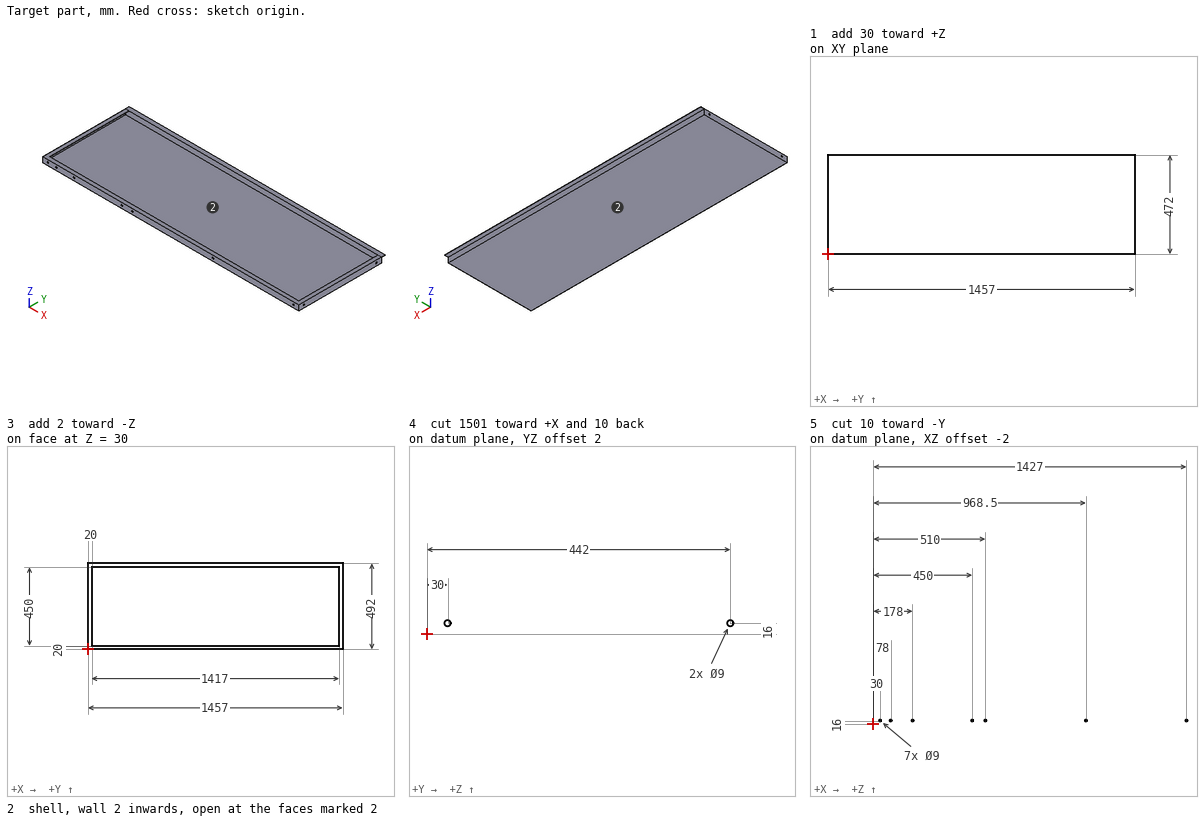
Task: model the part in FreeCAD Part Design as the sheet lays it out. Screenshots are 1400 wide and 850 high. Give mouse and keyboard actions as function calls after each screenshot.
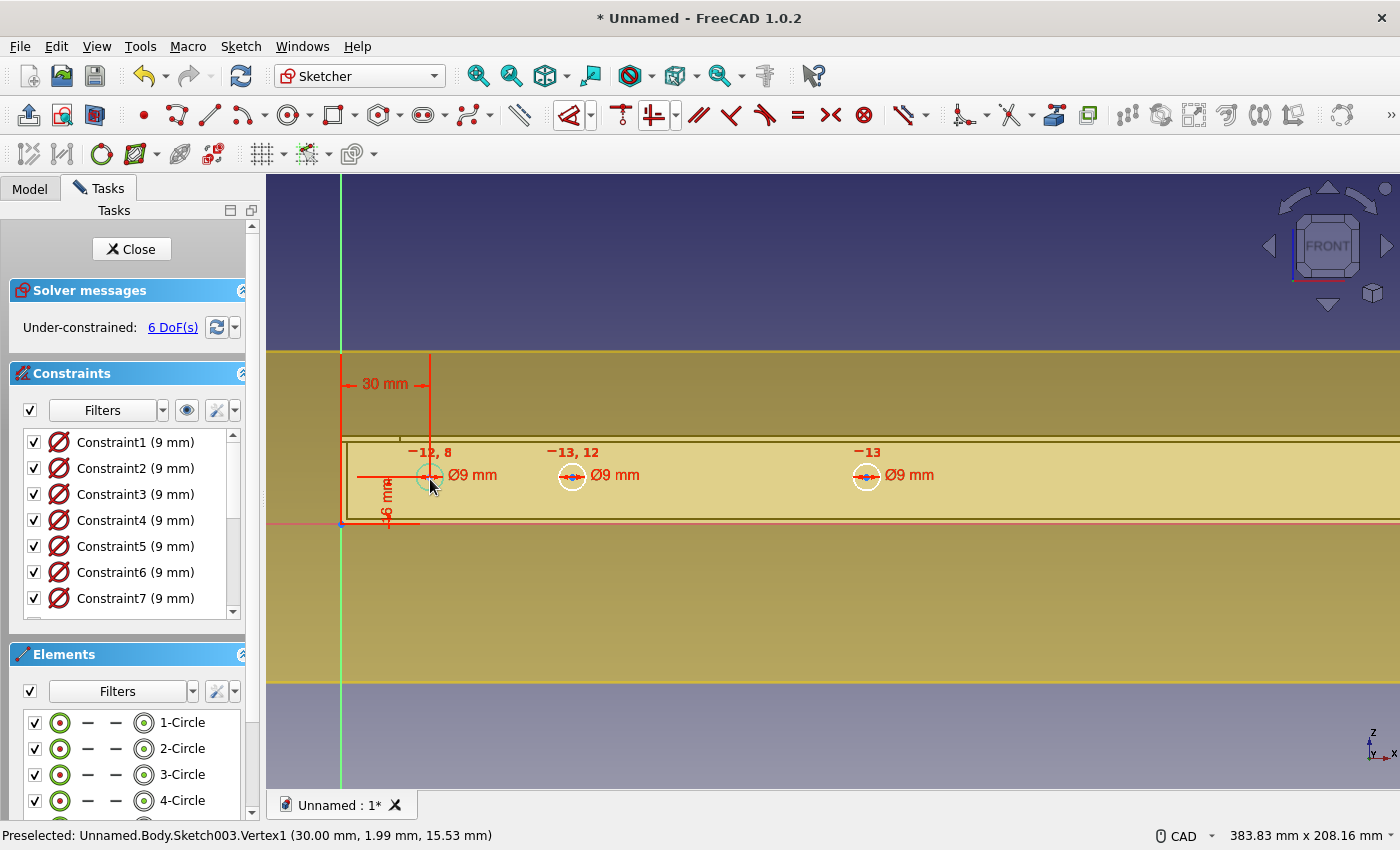
scroll(430, 479, down, 9)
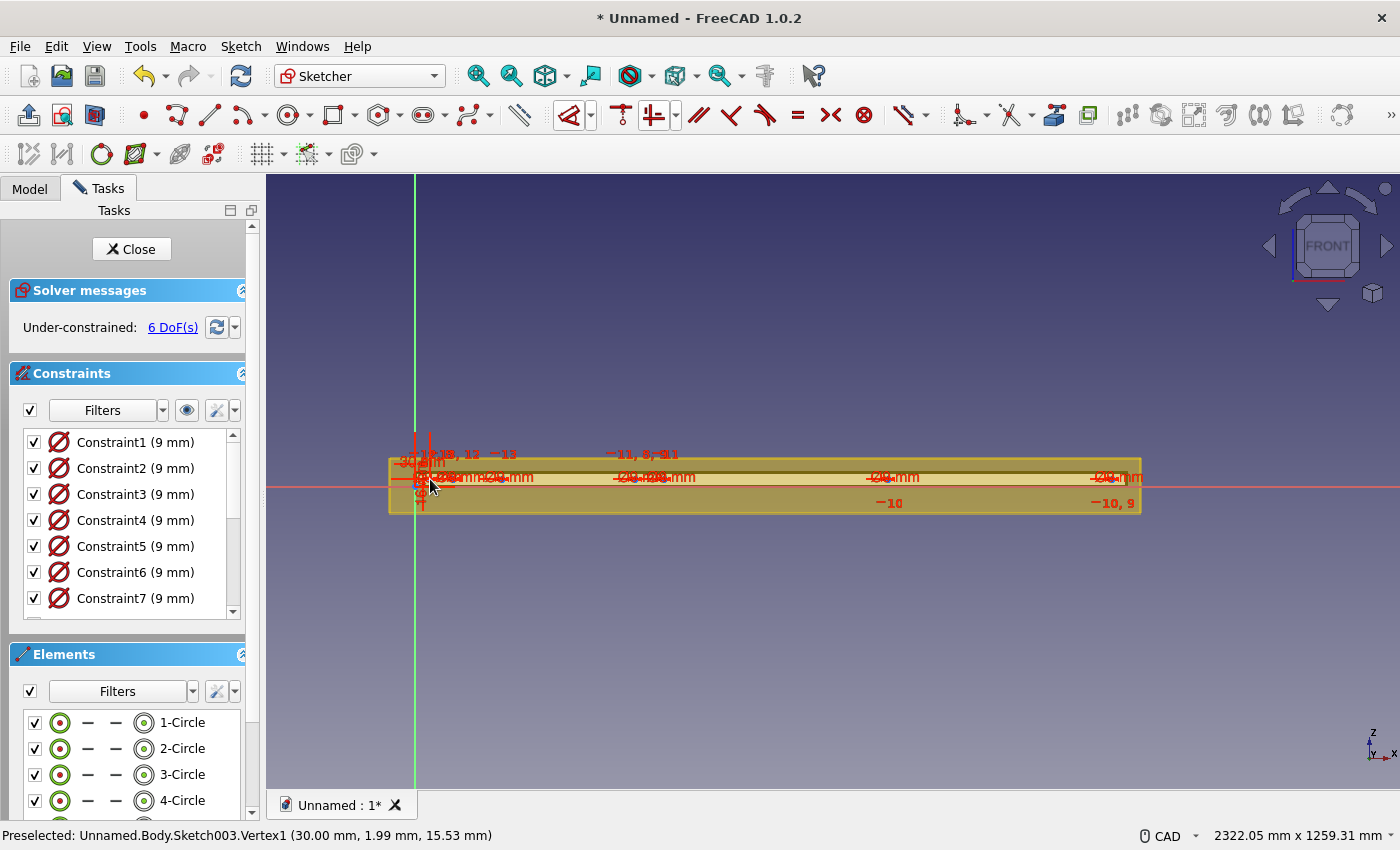
click(454, 479)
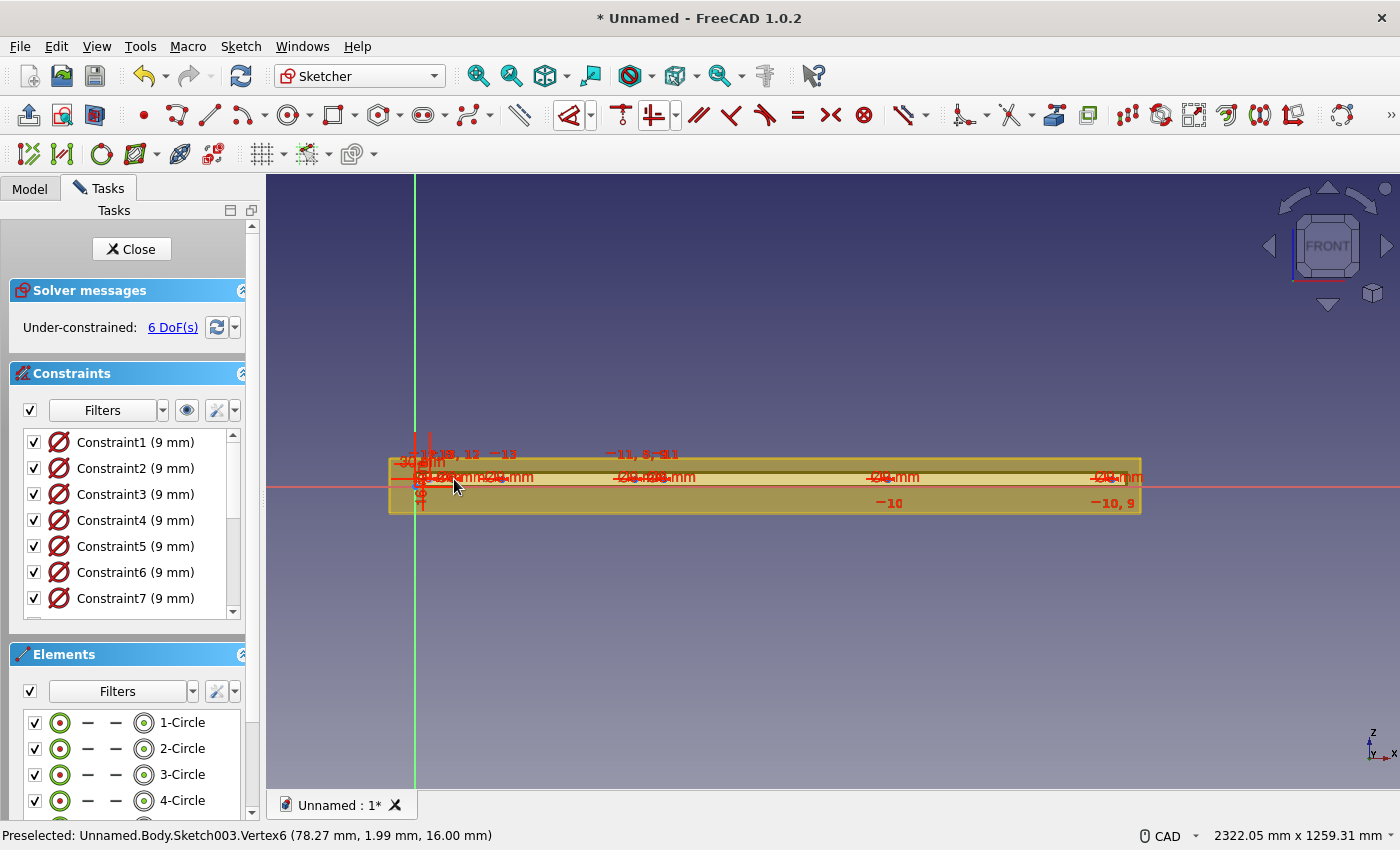
key(l)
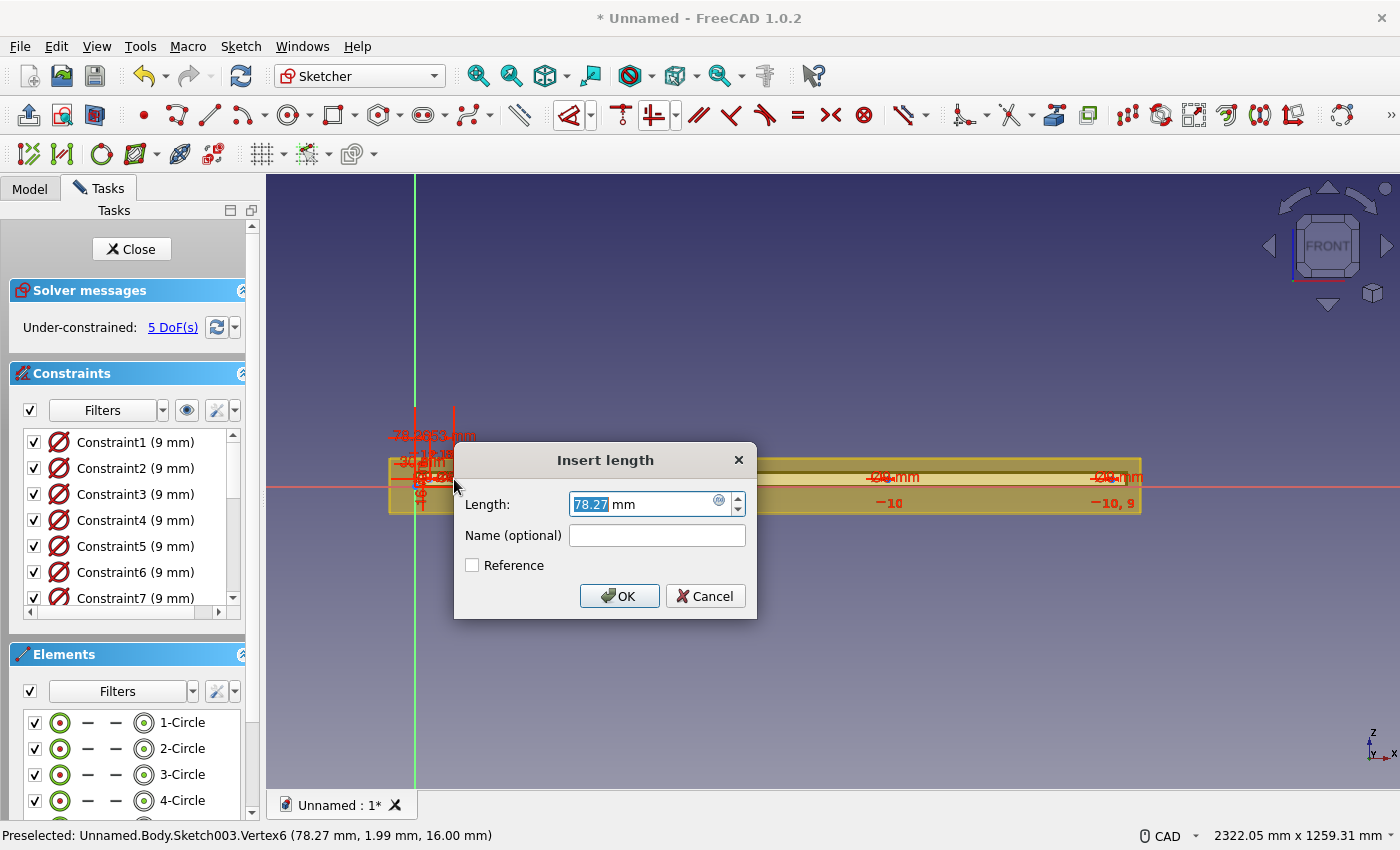
text(78)
key(Return)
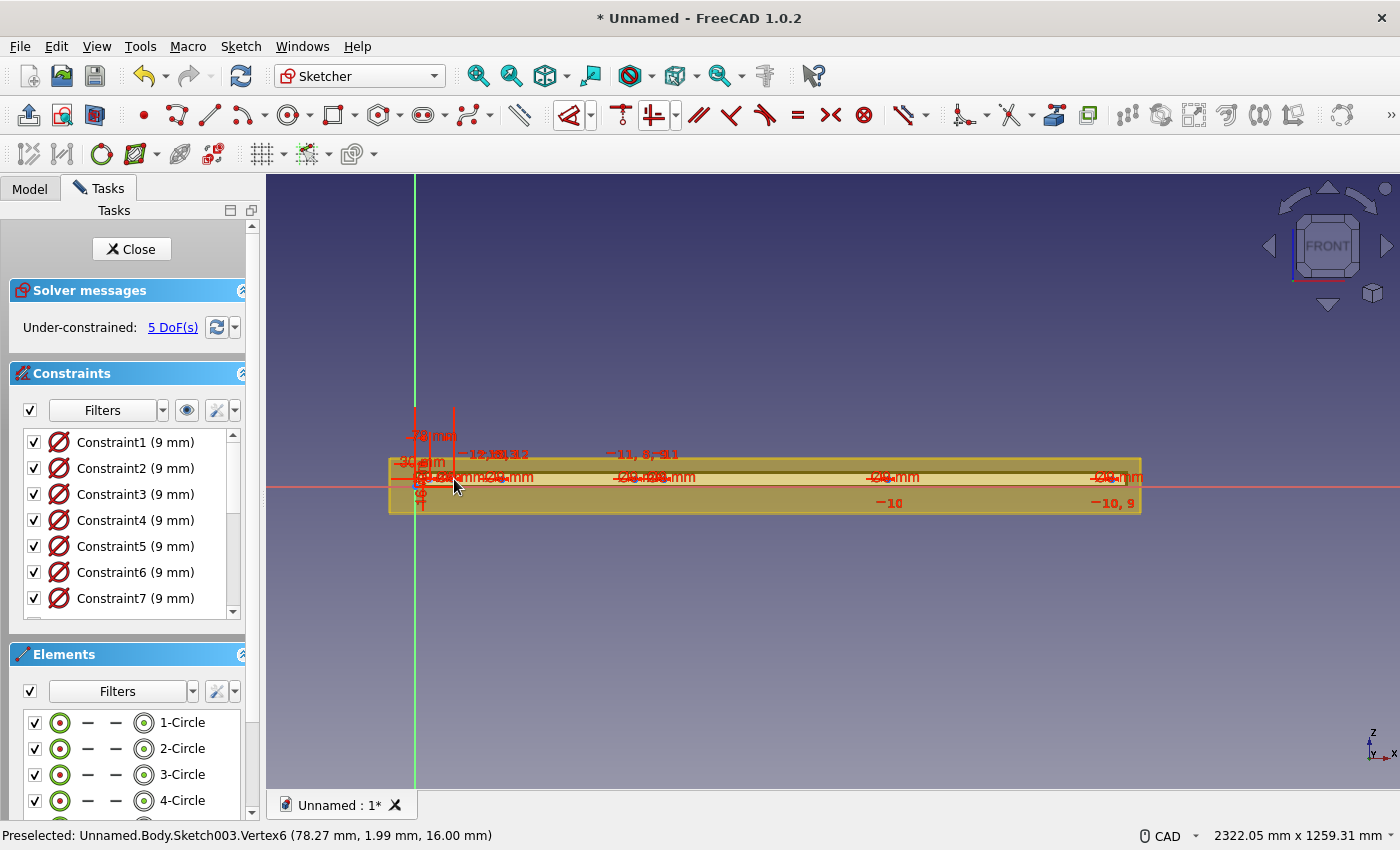
click(635, 479)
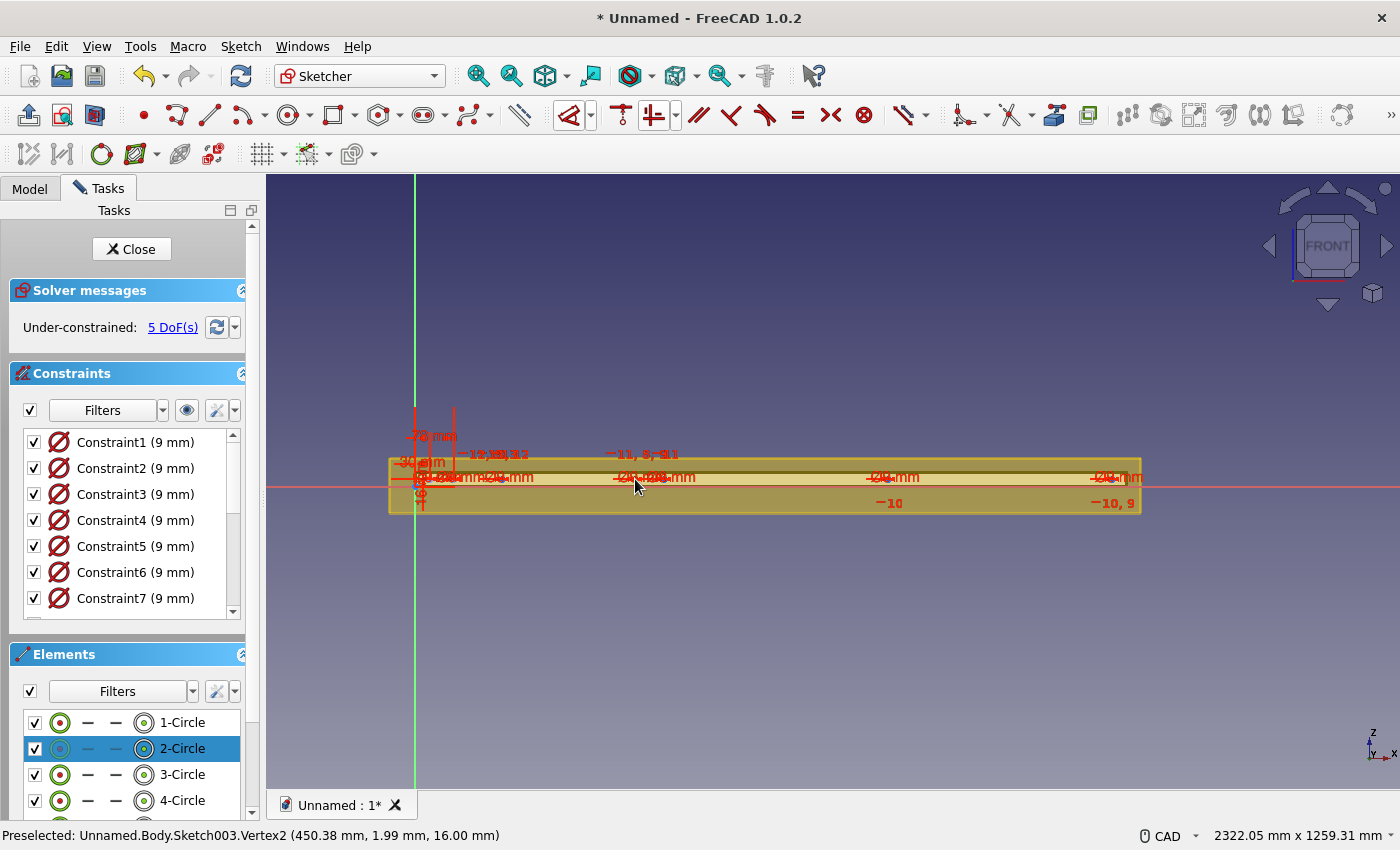
click(590, 116)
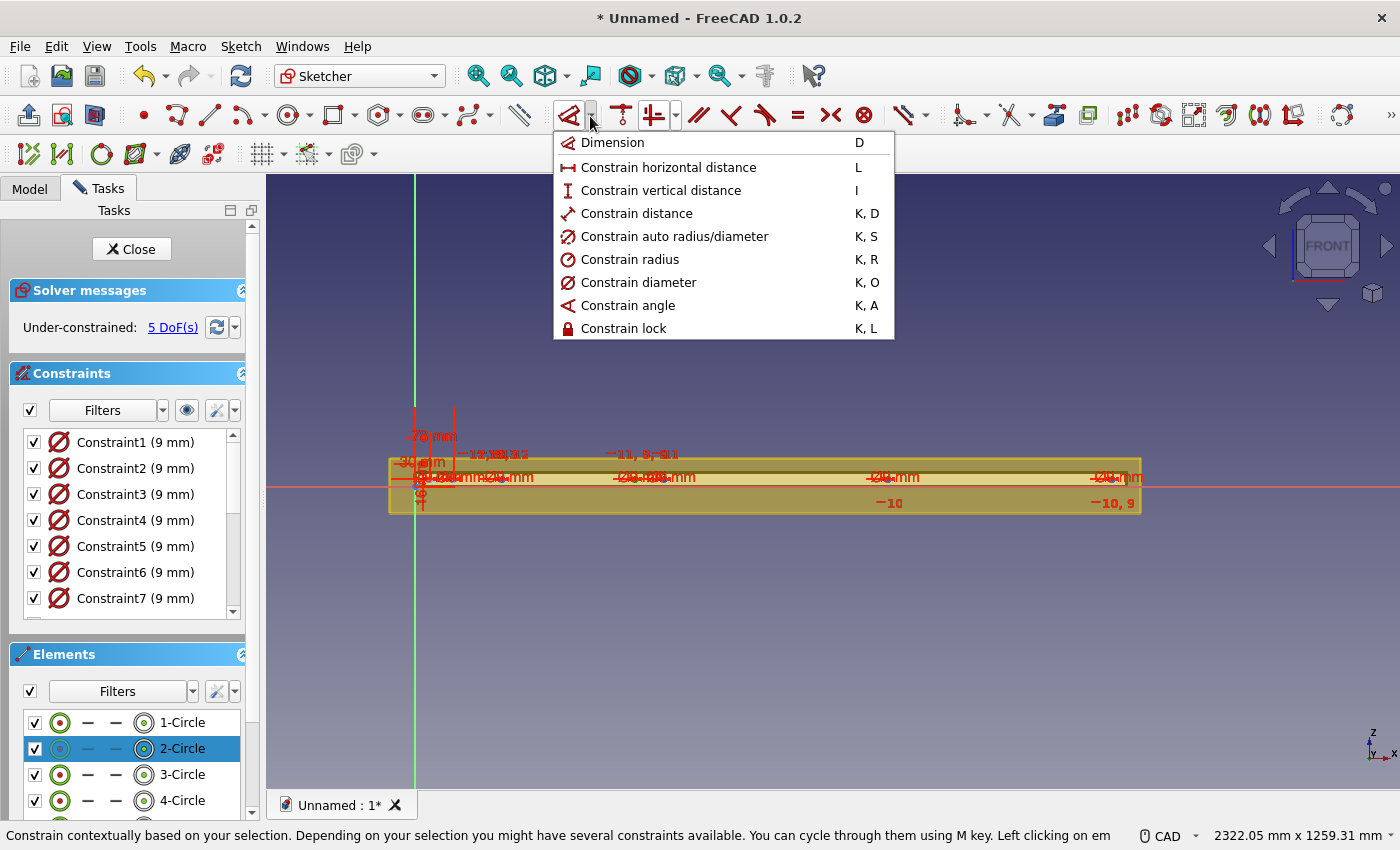
click(724, 168)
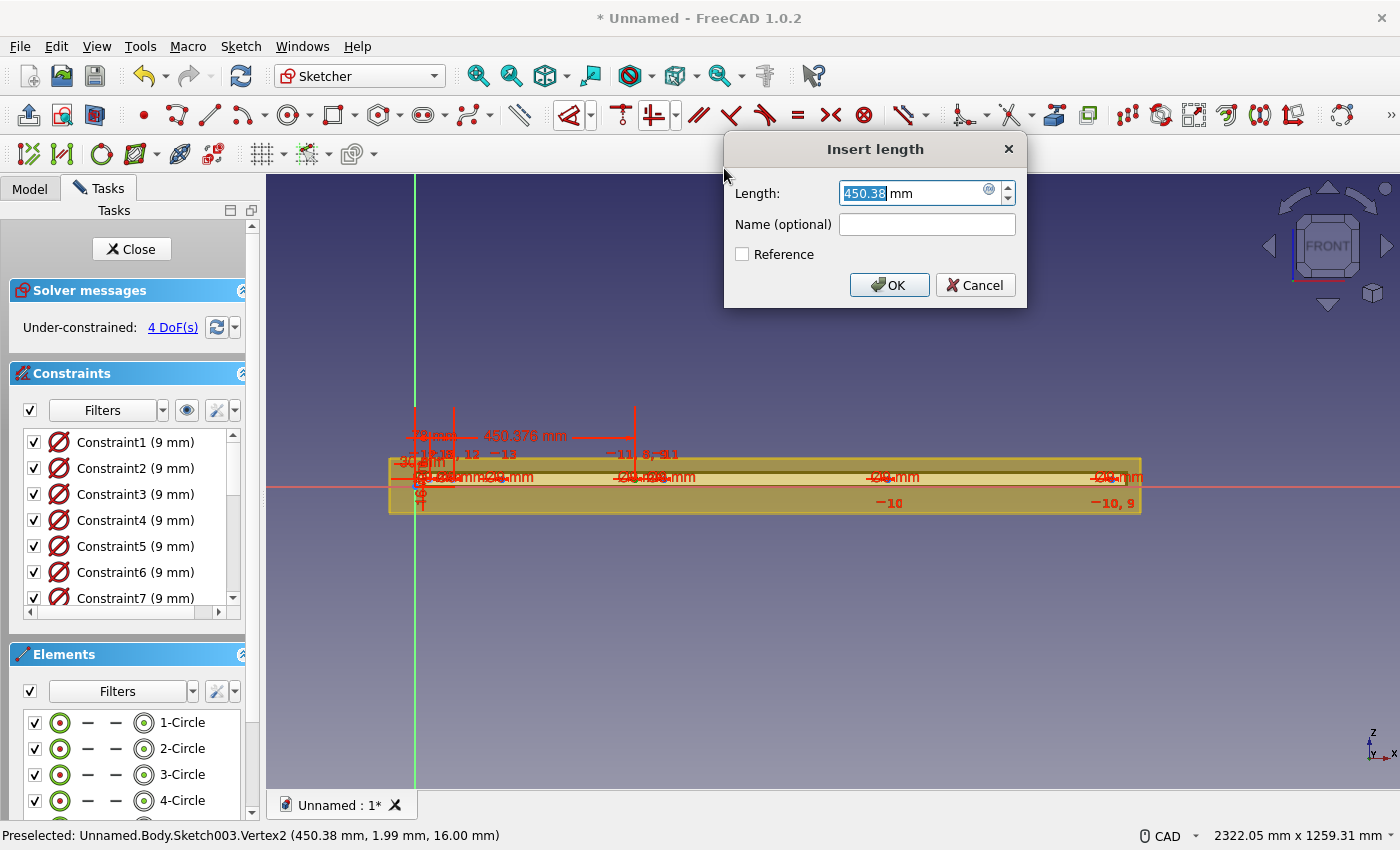
text(450)
key(Return)